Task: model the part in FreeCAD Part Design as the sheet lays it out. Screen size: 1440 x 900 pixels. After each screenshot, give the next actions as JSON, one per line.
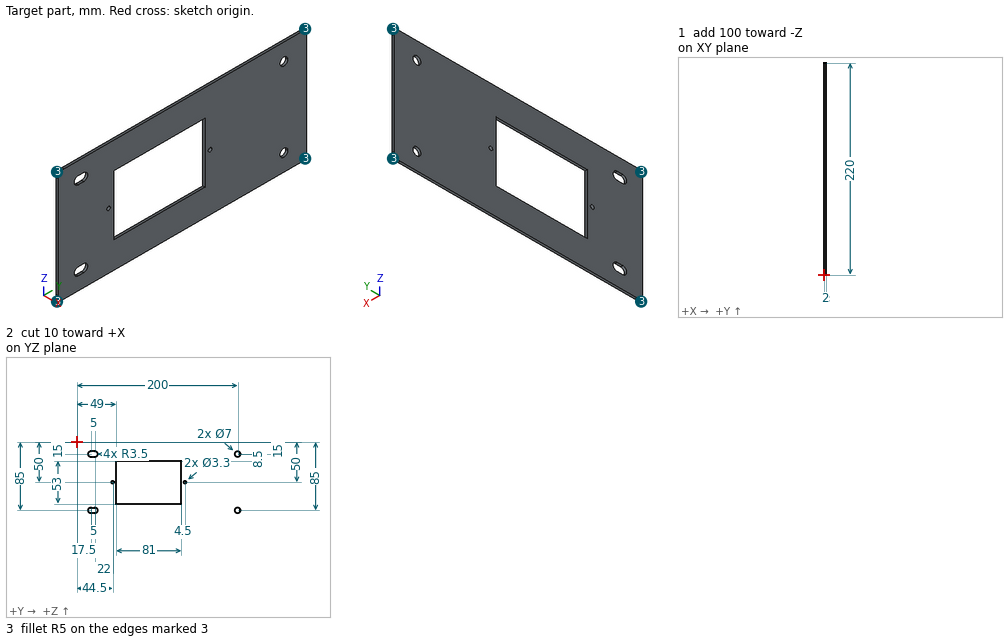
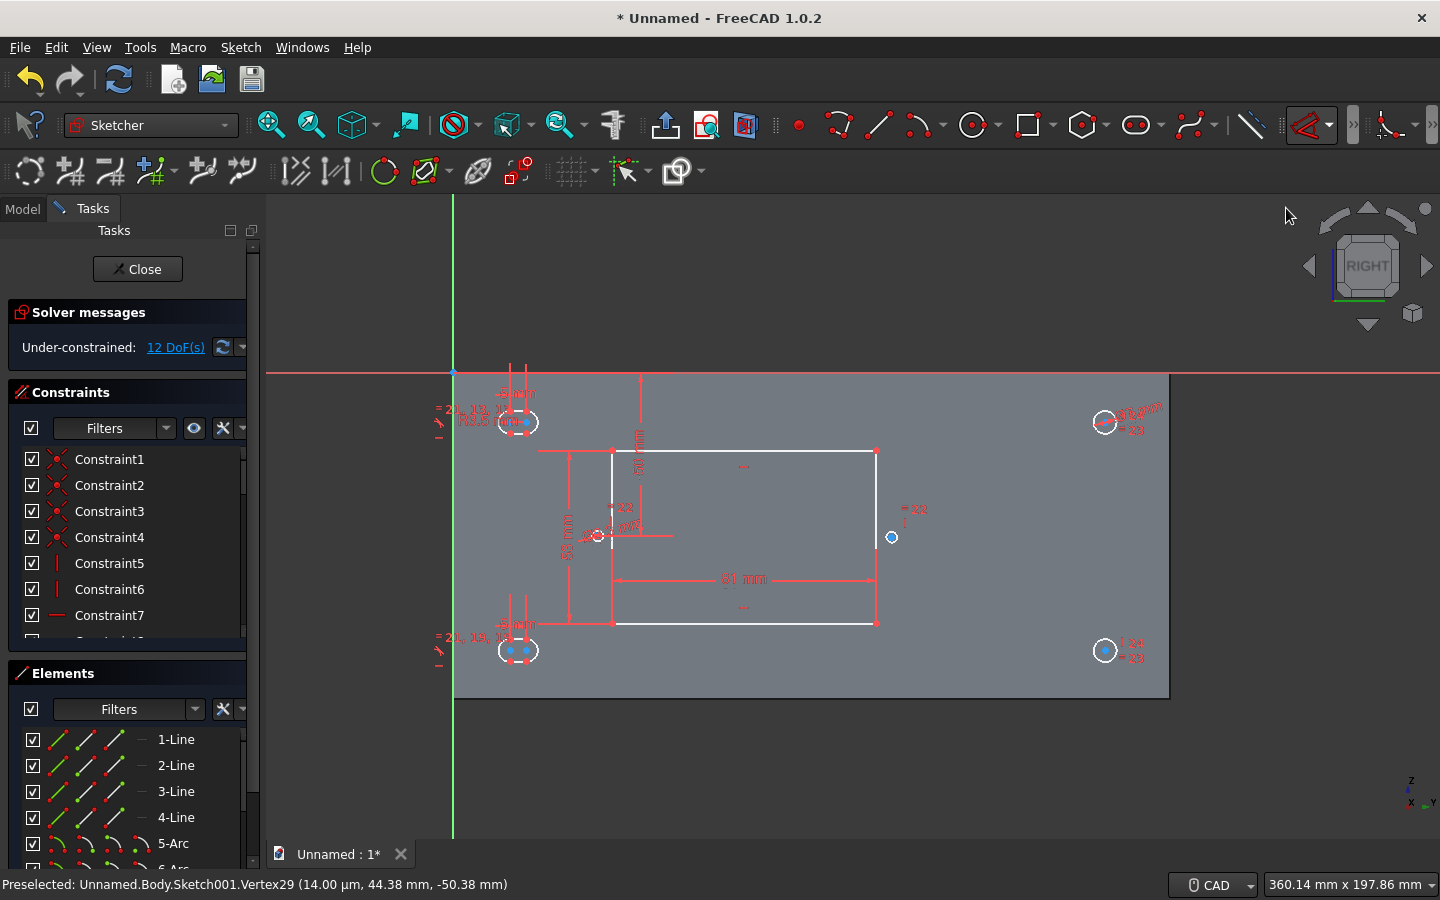
{"action": "left_click", "coordinate": [892, 537]}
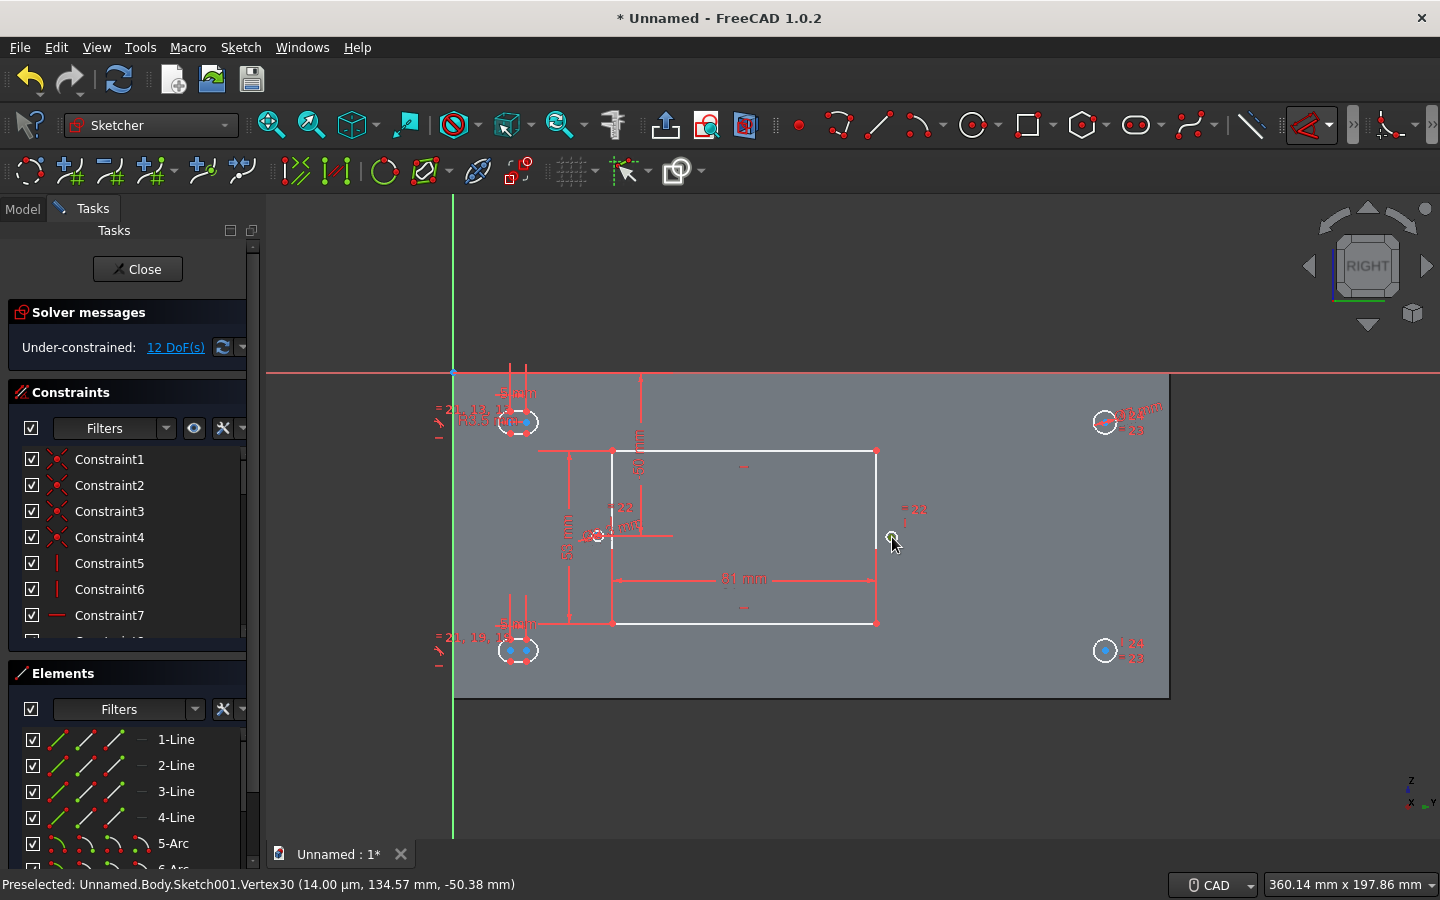
{"action": "key", "text": "i"}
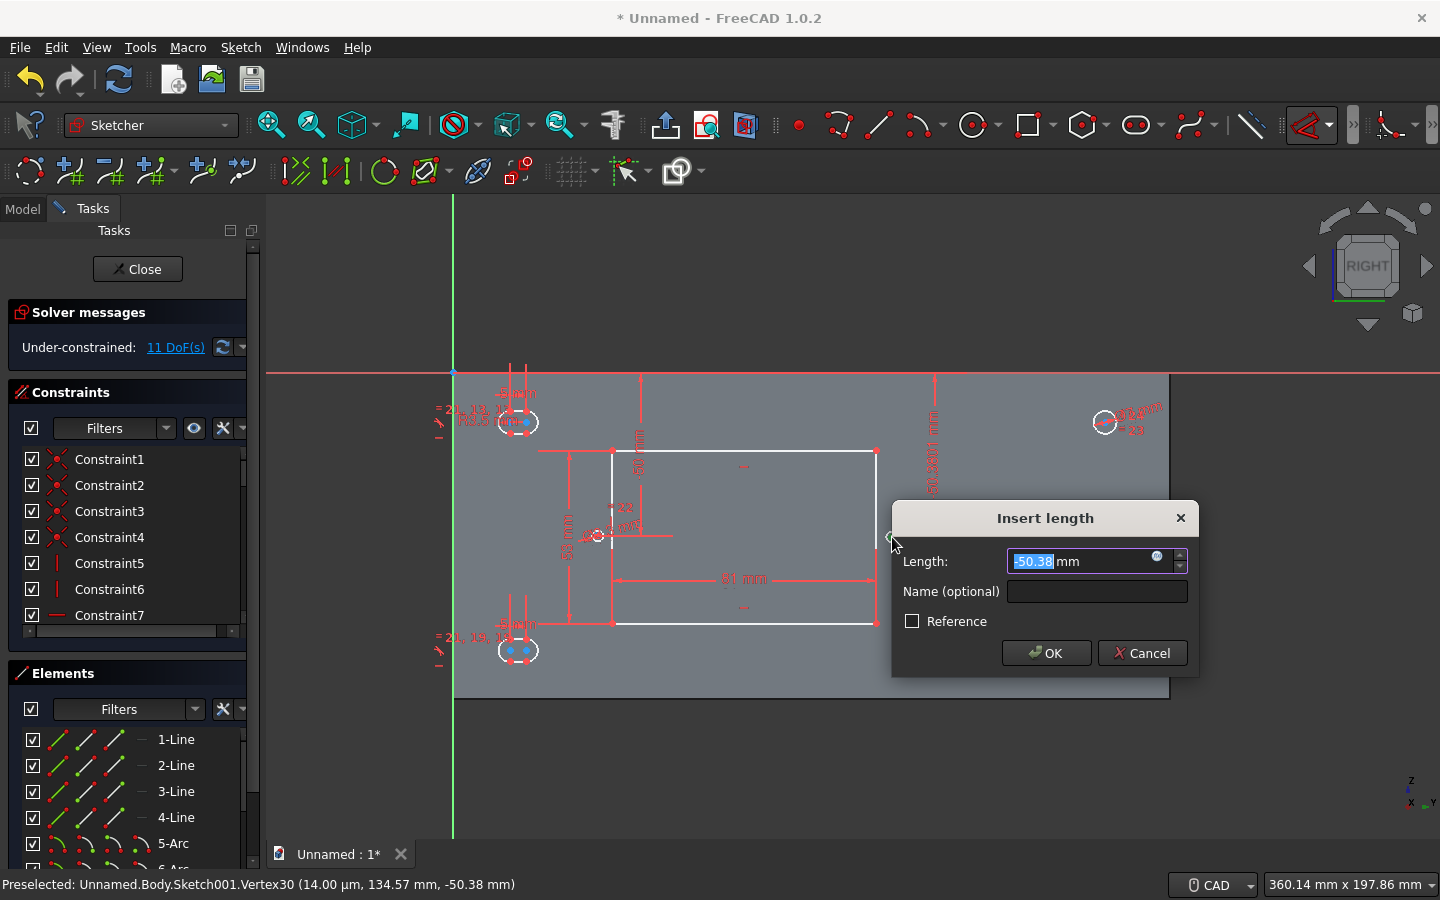
{"action": "type", "text": "-50"}
{"action": "key", "text": "Return"}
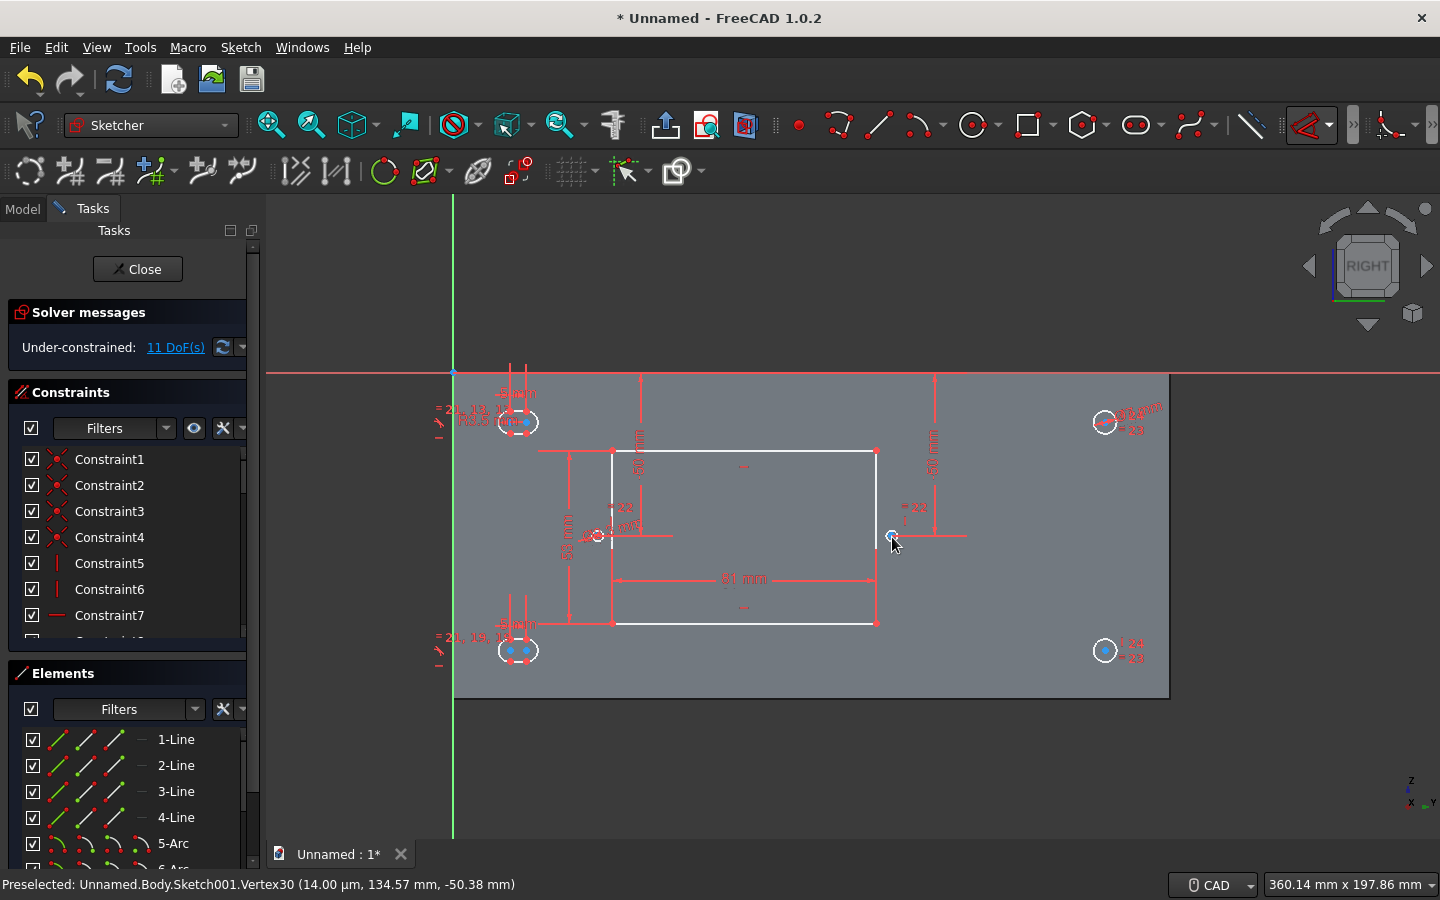
{"action": "left_click", "coordinate": [1105, 422]}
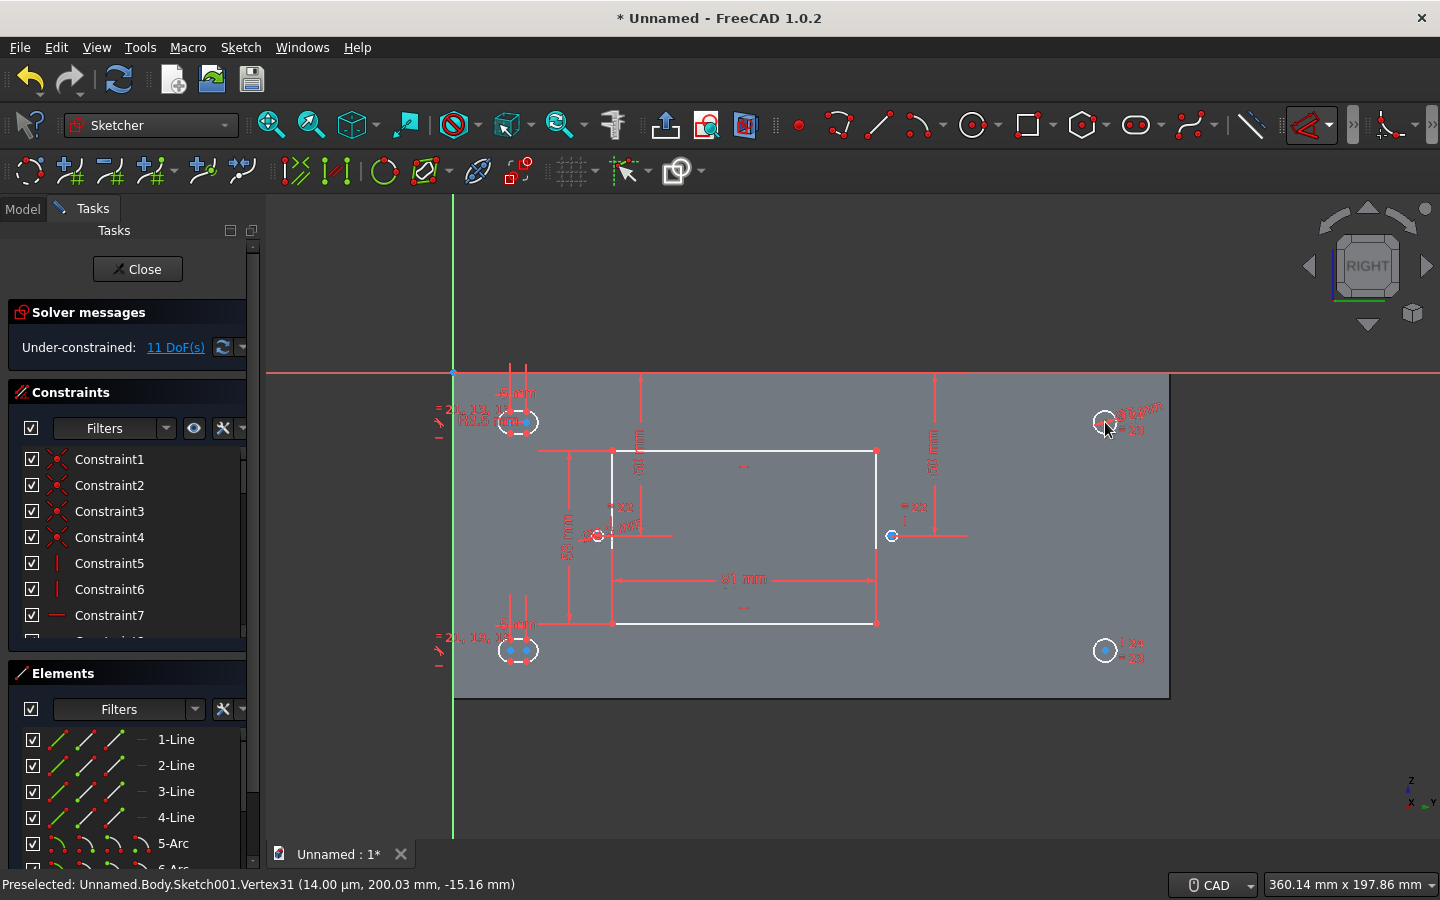
{"action": "left_click", "coordinate": [1332, 126]}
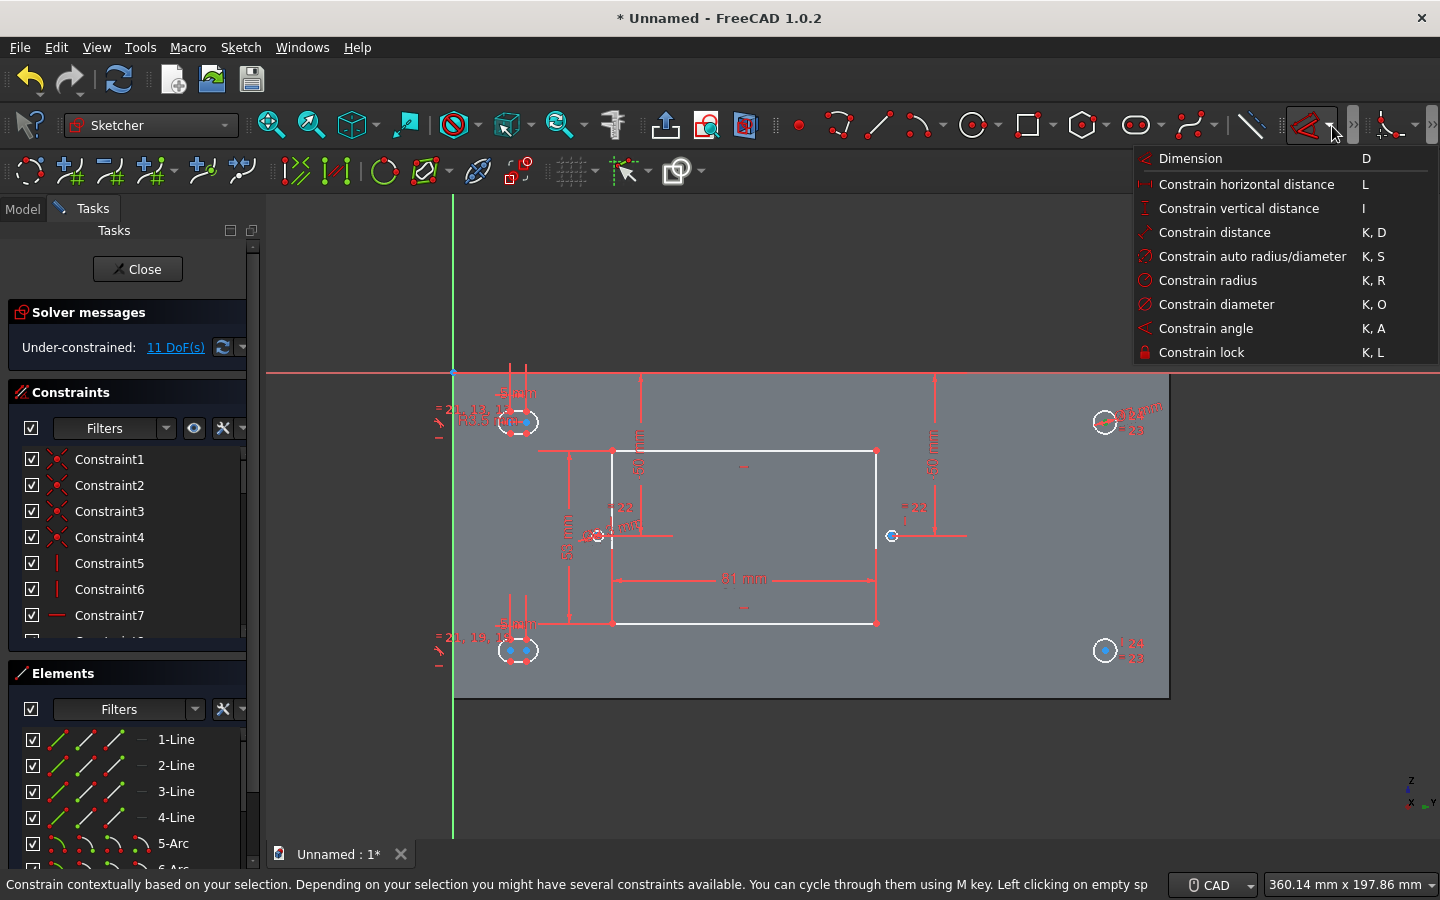
{"action": "left_click", "coordinate": [1286, 208]}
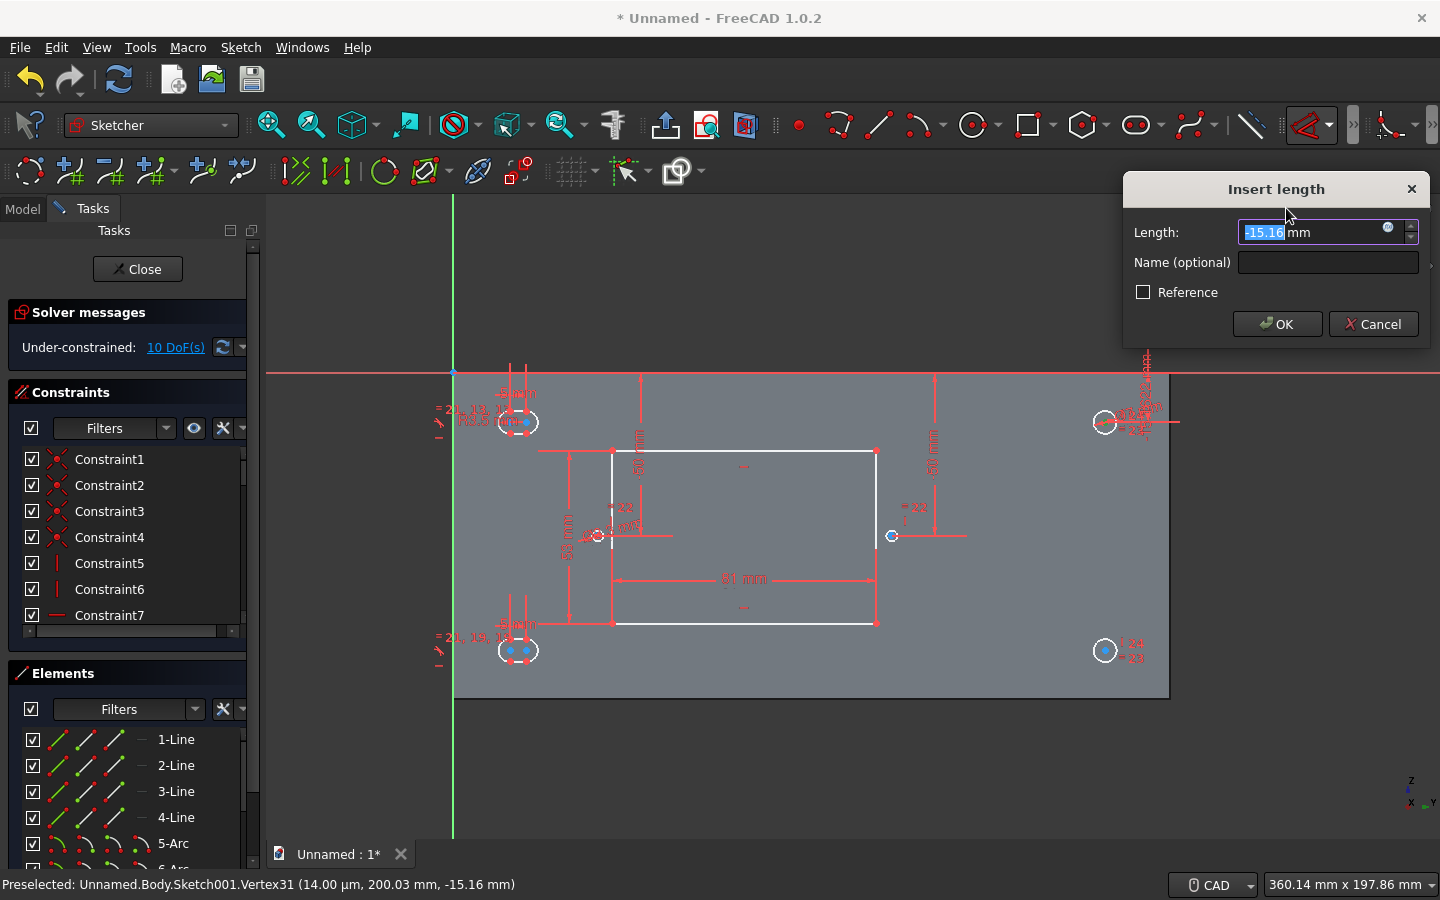
{"action": "type", "text": "-15"}
{"action": "key", "text": "Return"}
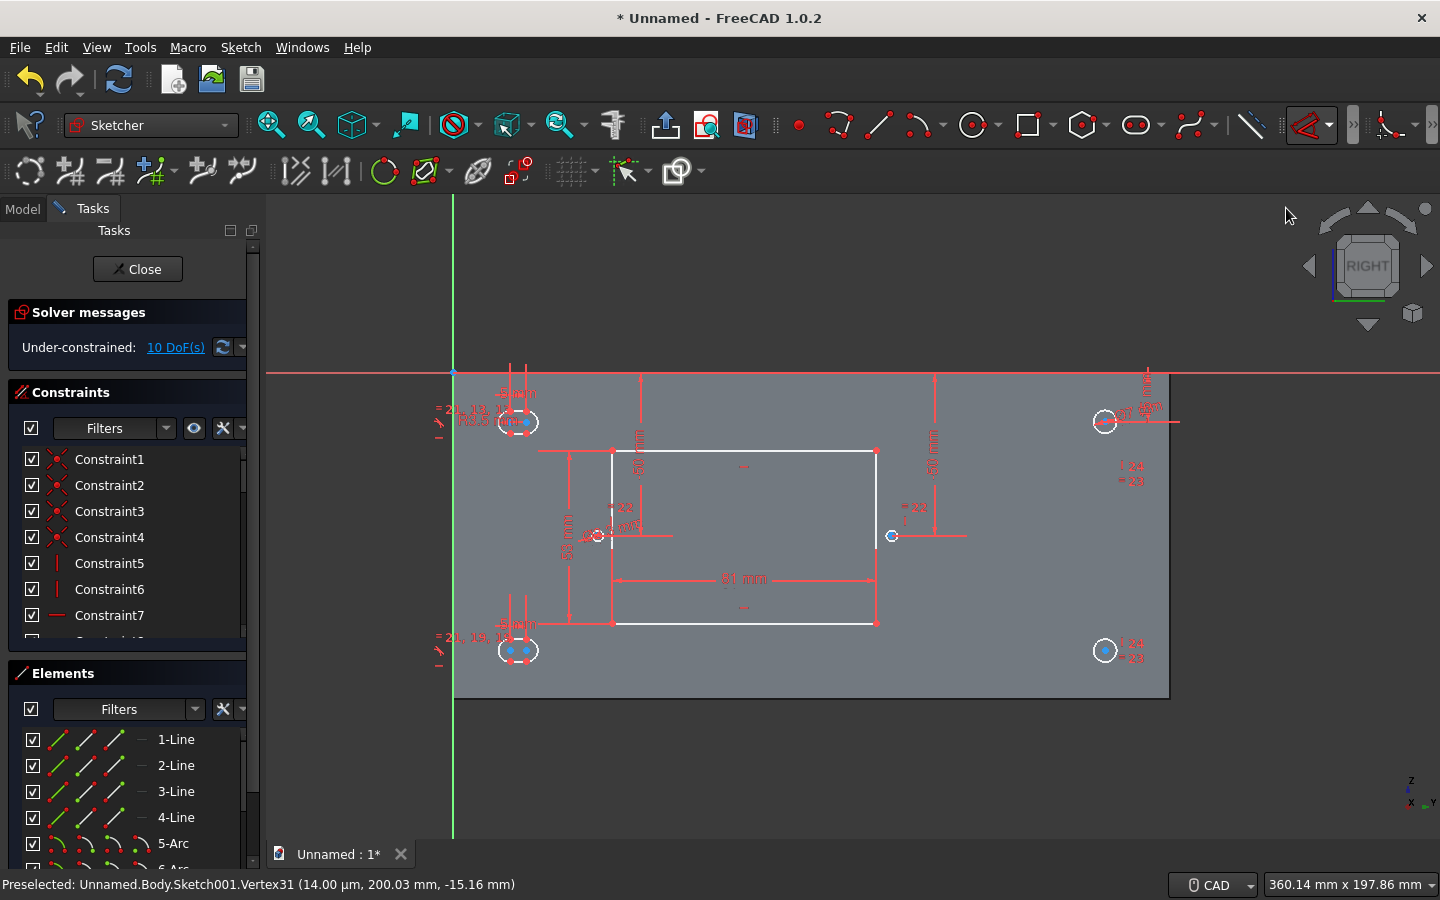
{"action": "left_click", "coordinate": [1105, 651]}